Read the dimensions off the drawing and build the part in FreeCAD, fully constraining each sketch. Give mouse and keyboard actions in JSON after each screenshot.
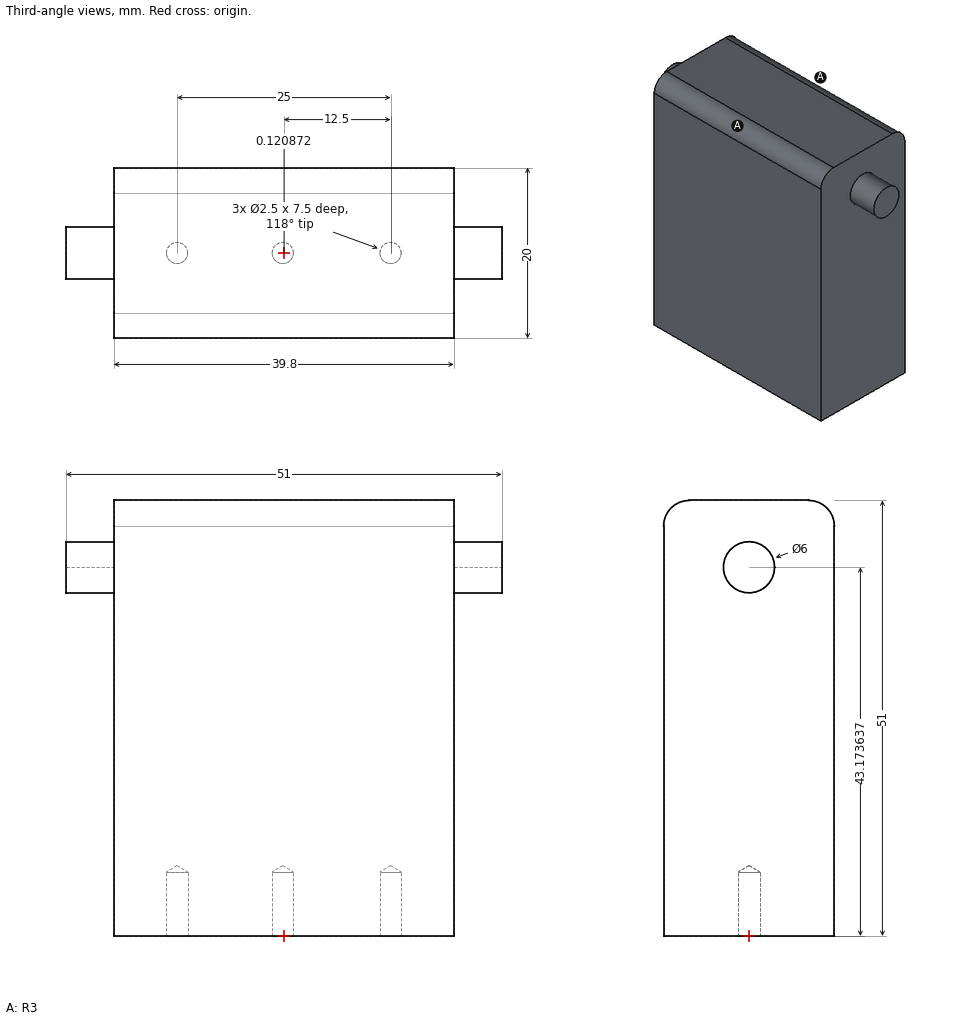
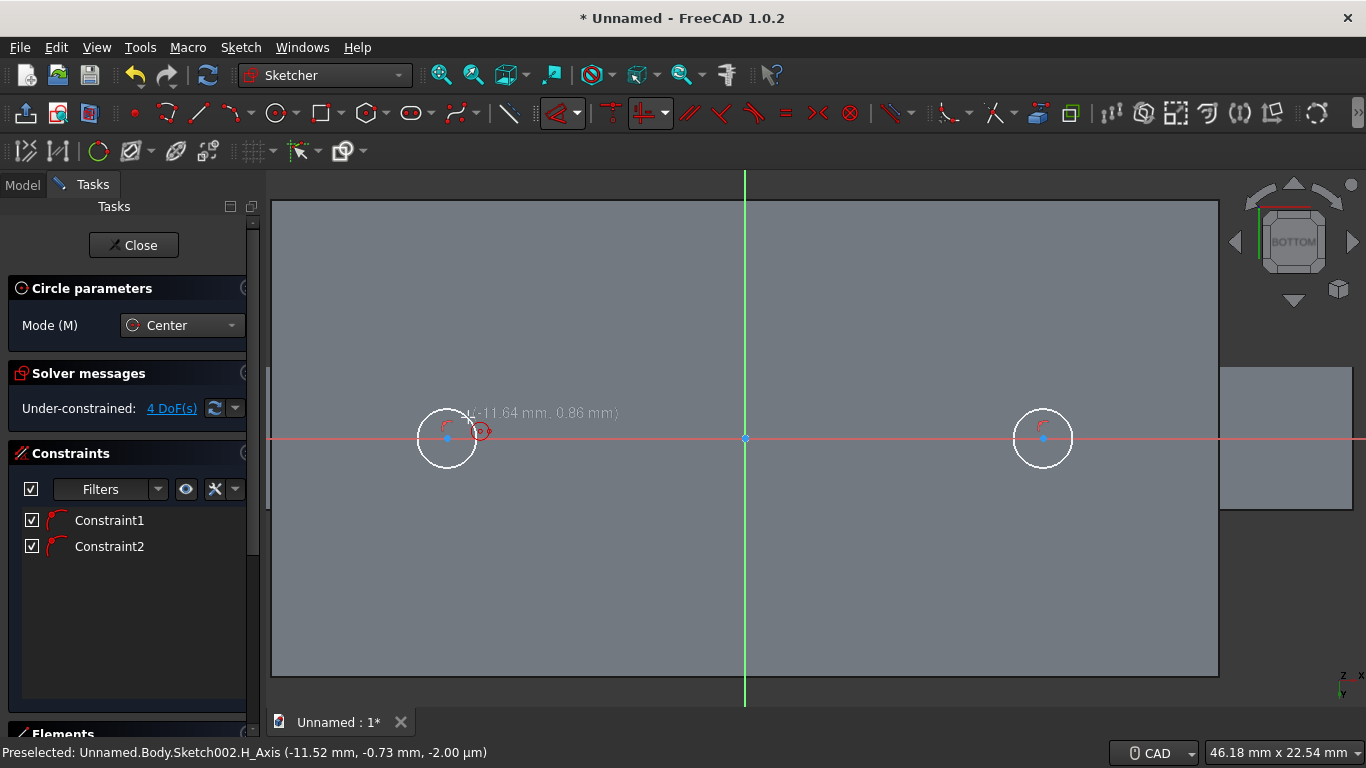
{"action": "scroll", "coordinate": [742, 438], "scroll_direction": "up", "scroll_amount": 9}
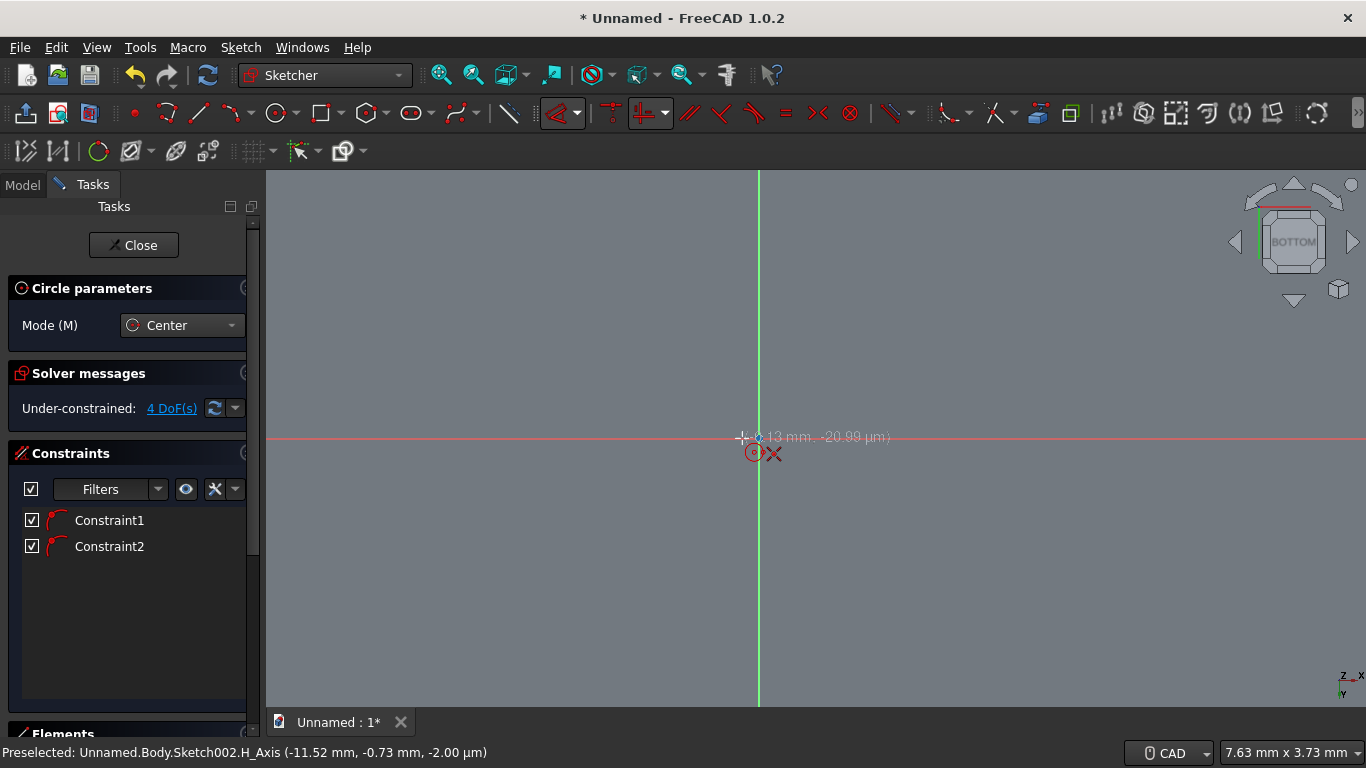
{"action": "left_click", "coordinate": [742, 438]}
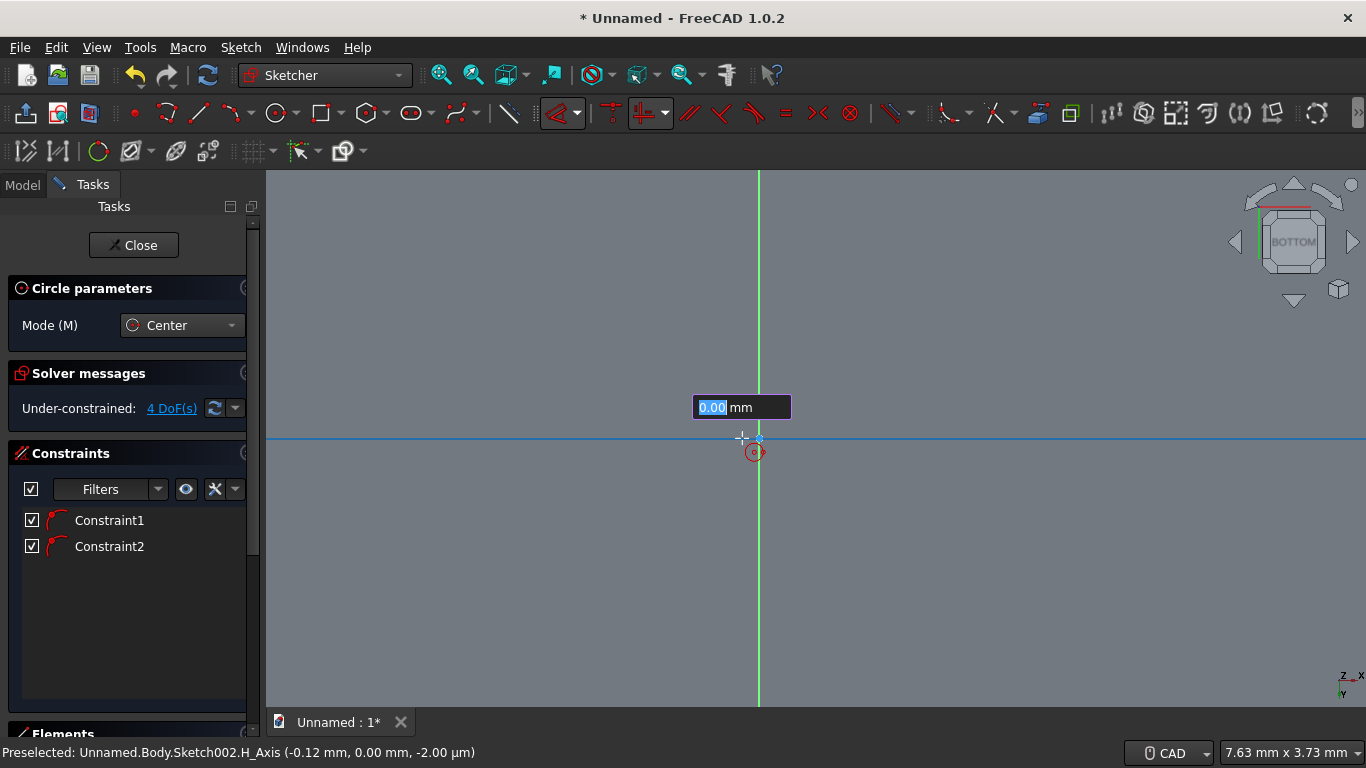
{"action": "scroll", "coordinate": [745, 438], "scroll_direction": "down", "scroll_amount": 9}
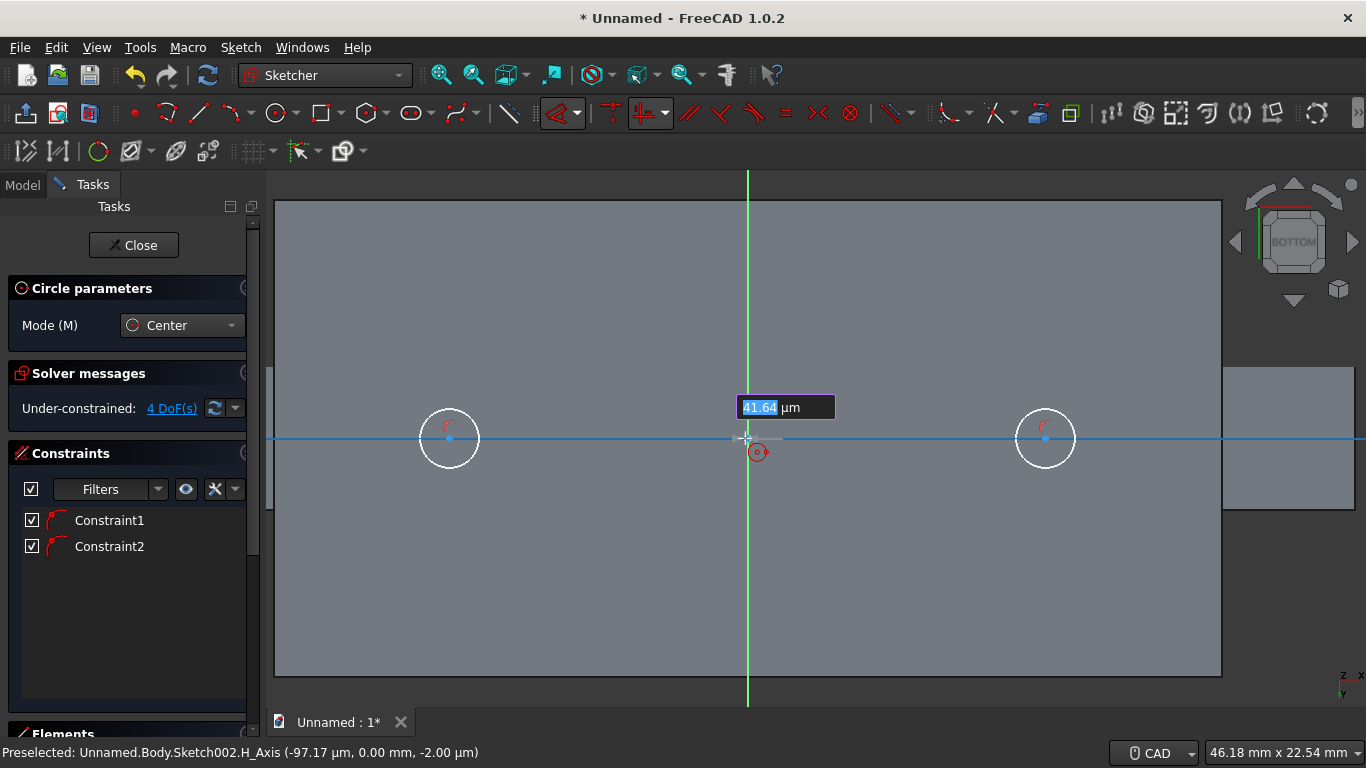
{"action": "left_click", "coordinate": [766, 417]}
{"action": "key", "text": "Escape"}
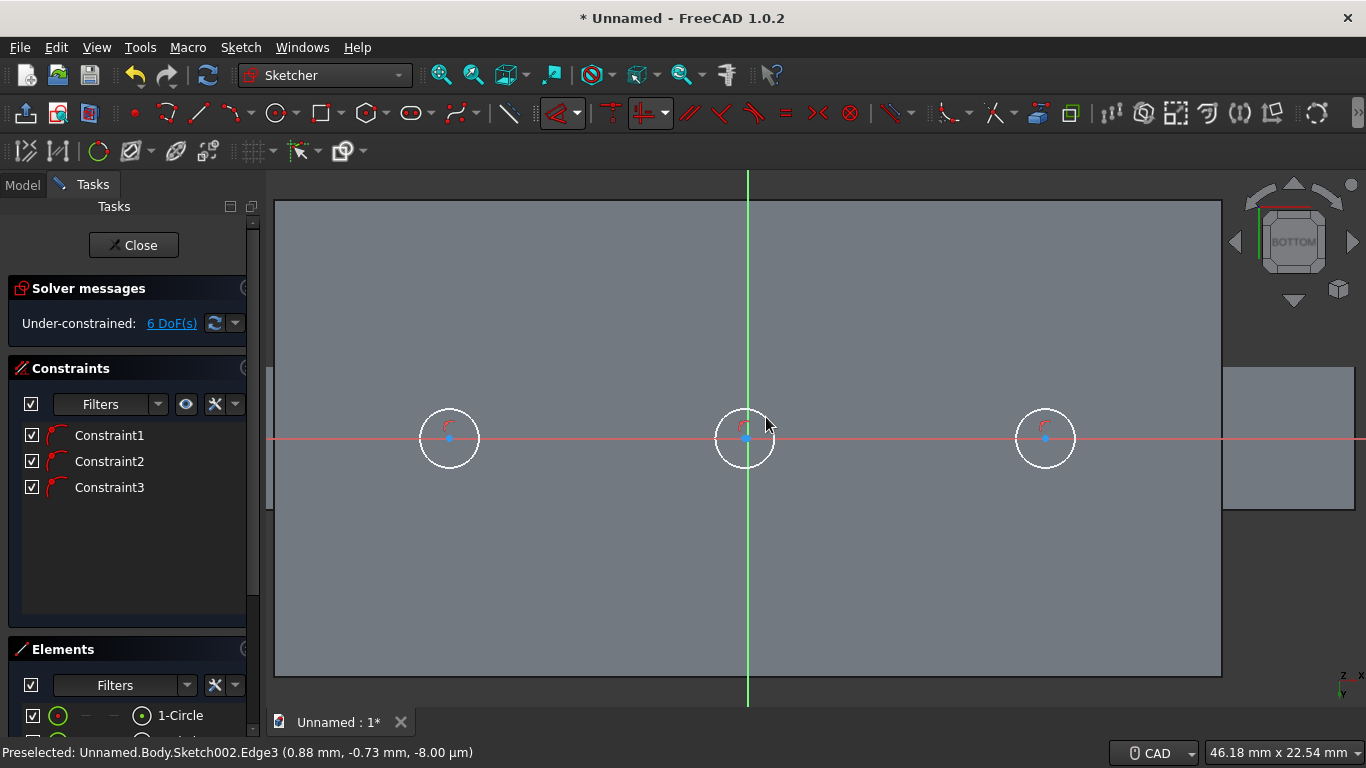
{"action": "left_click", "coordinate": [1066, 418]}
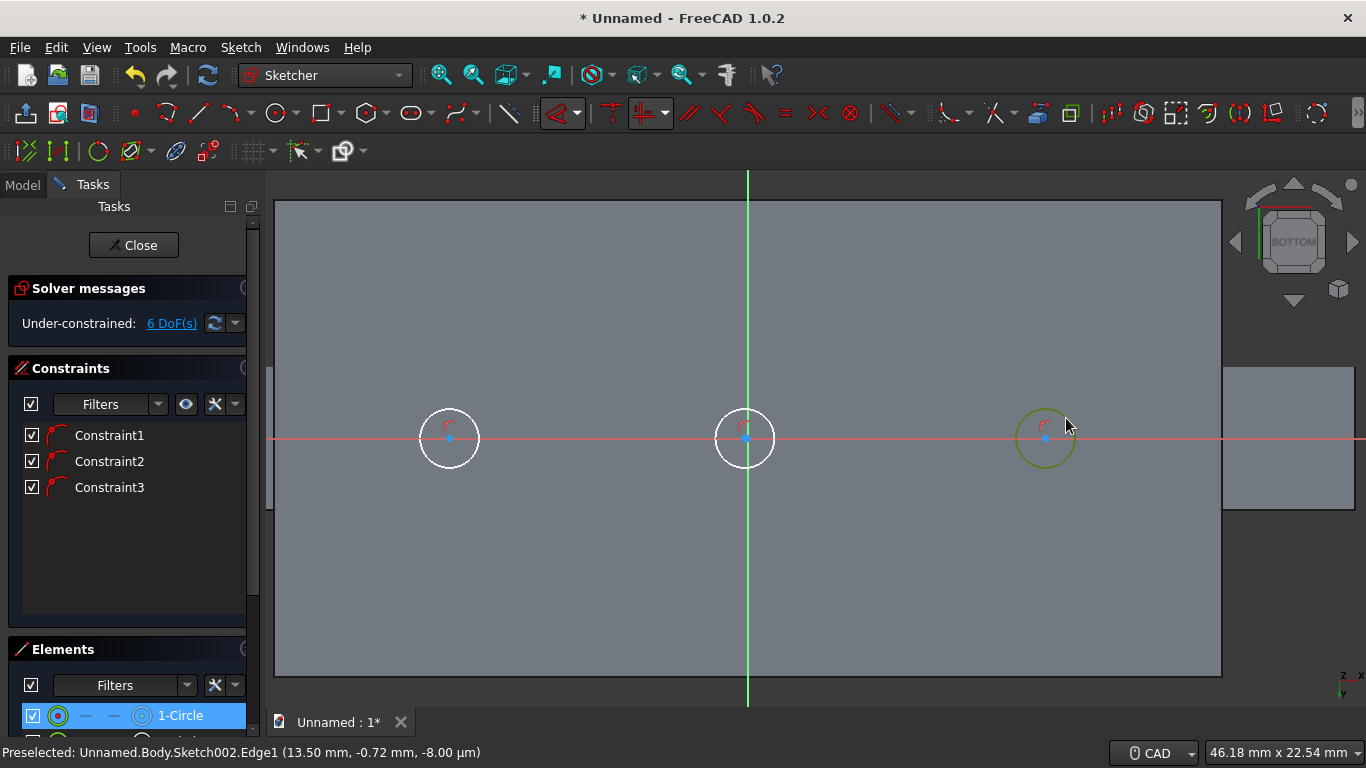
{"action": "left_click", "coordinate": [470, 418]}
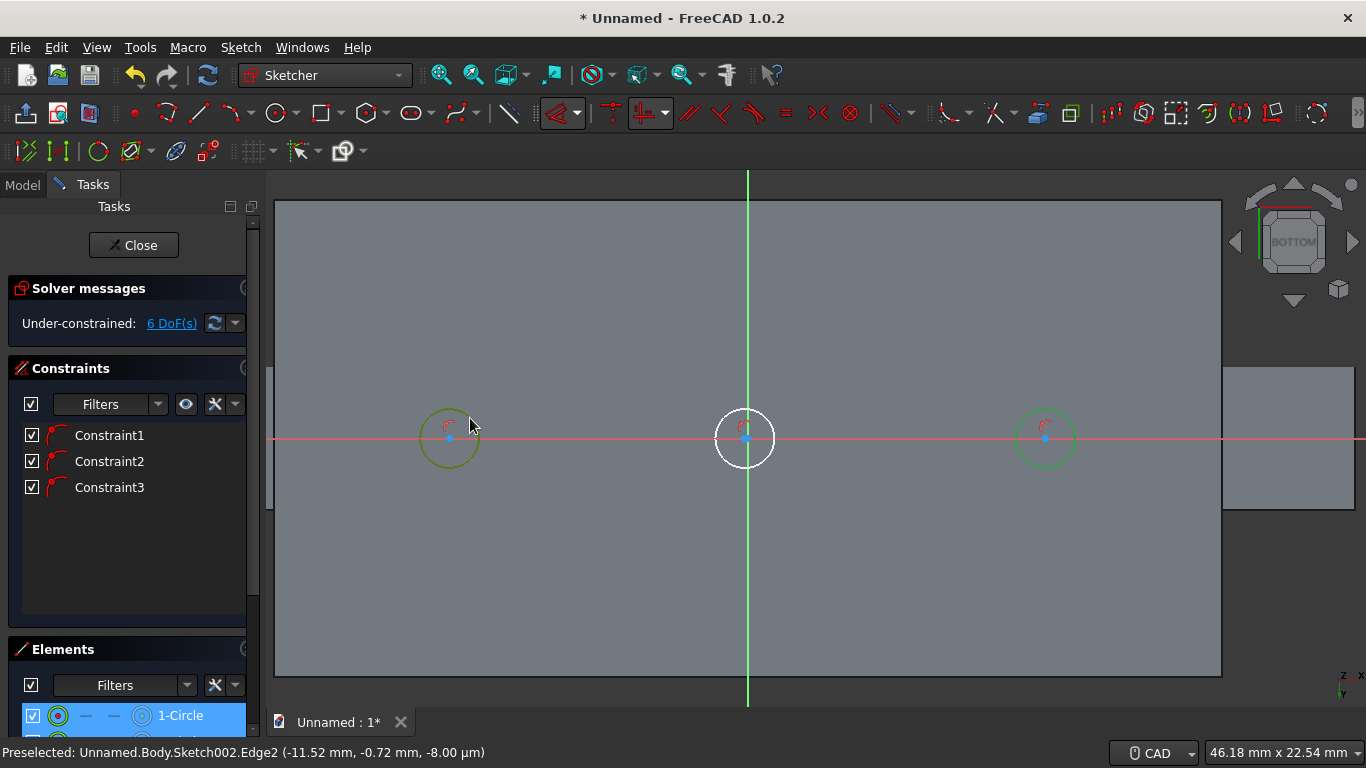
{"action": "left_click", "coordinate": [766, 418]}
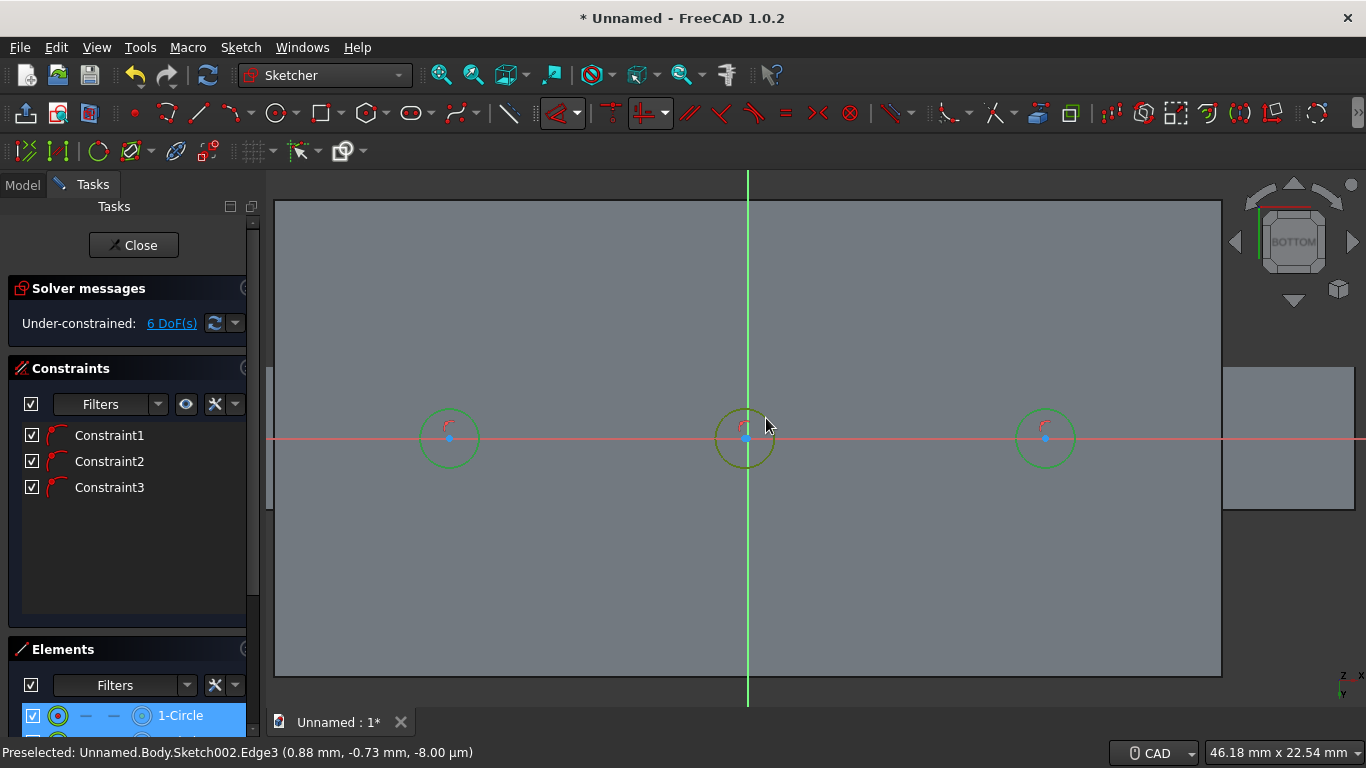
{"action": "left_click", "coordinate": [786, 114]}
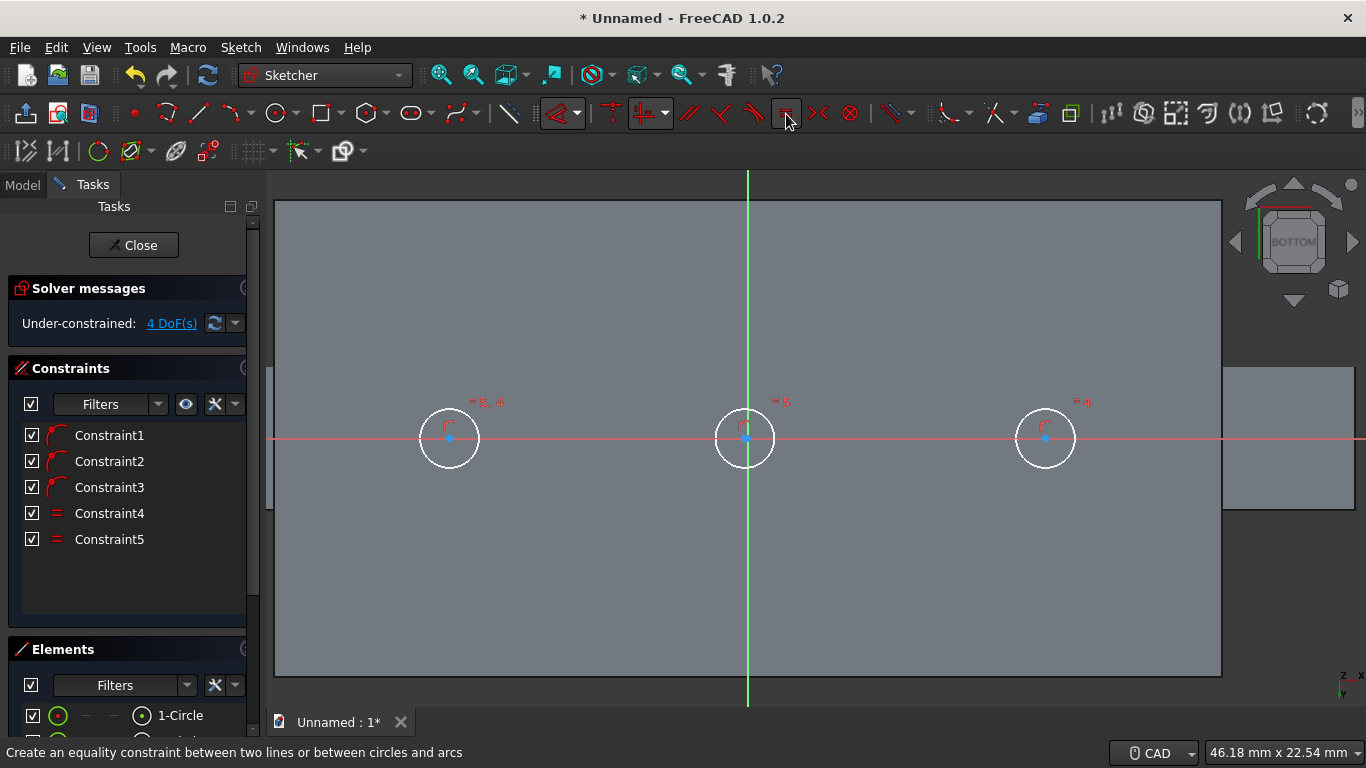
{"action": "left_click", "coordinate": [1066, 418]}